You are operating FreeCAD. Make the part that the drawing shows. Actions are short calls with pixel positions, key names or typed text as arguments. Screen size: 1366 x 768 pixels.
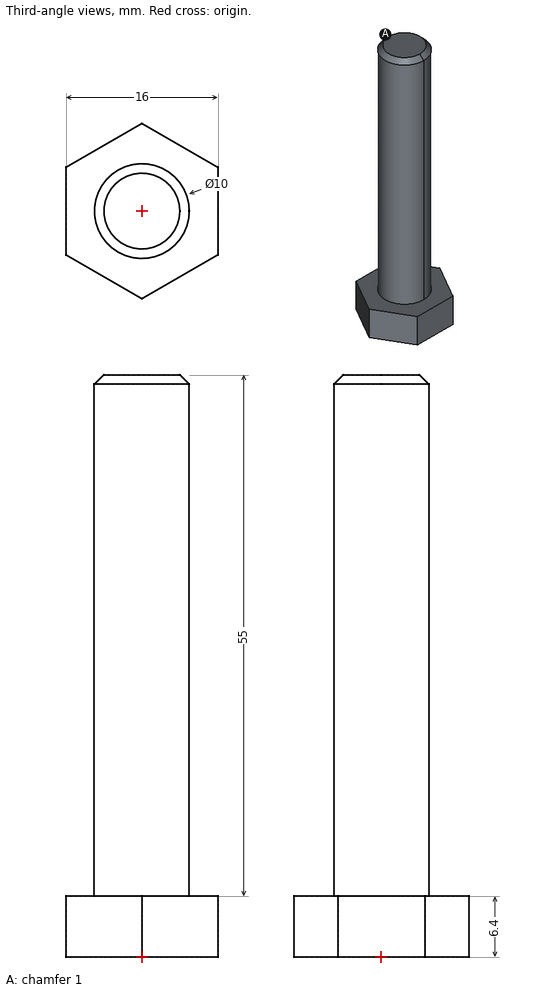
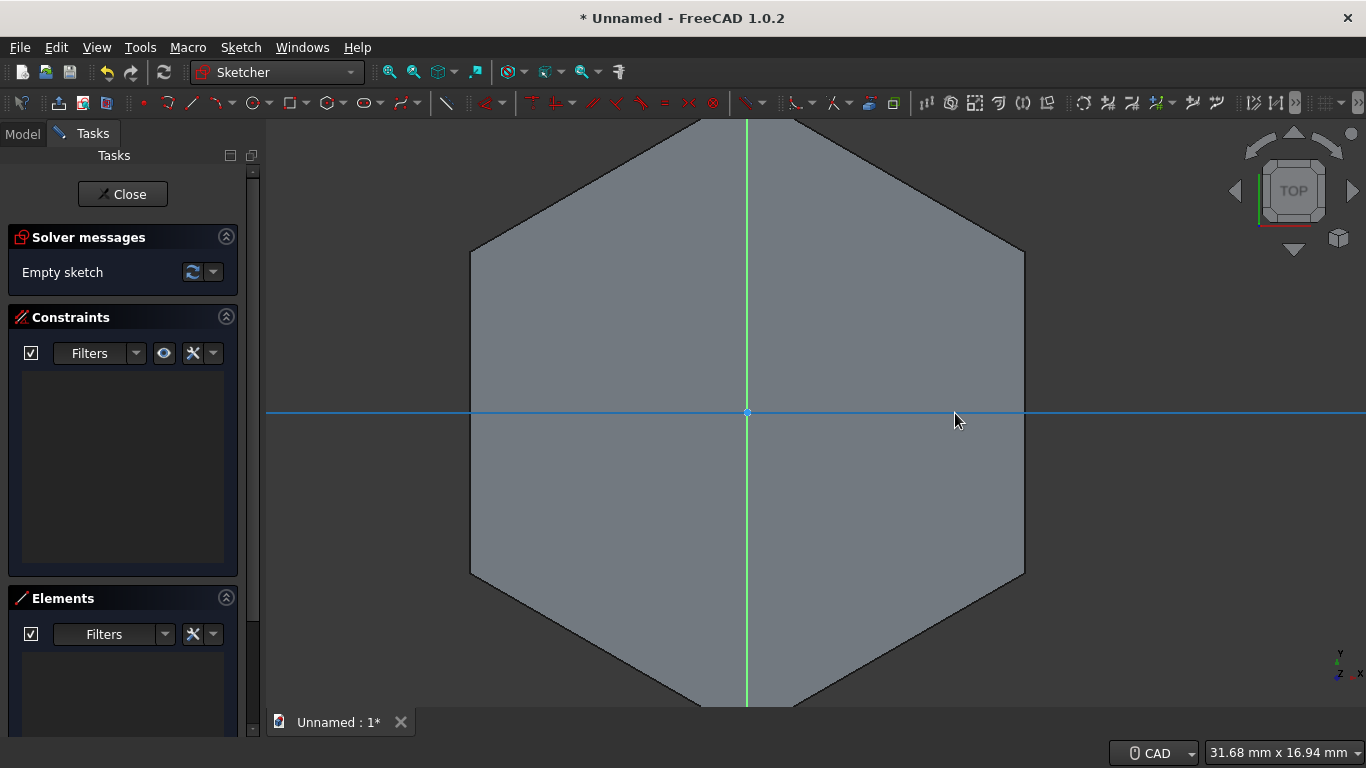
click(254, 104)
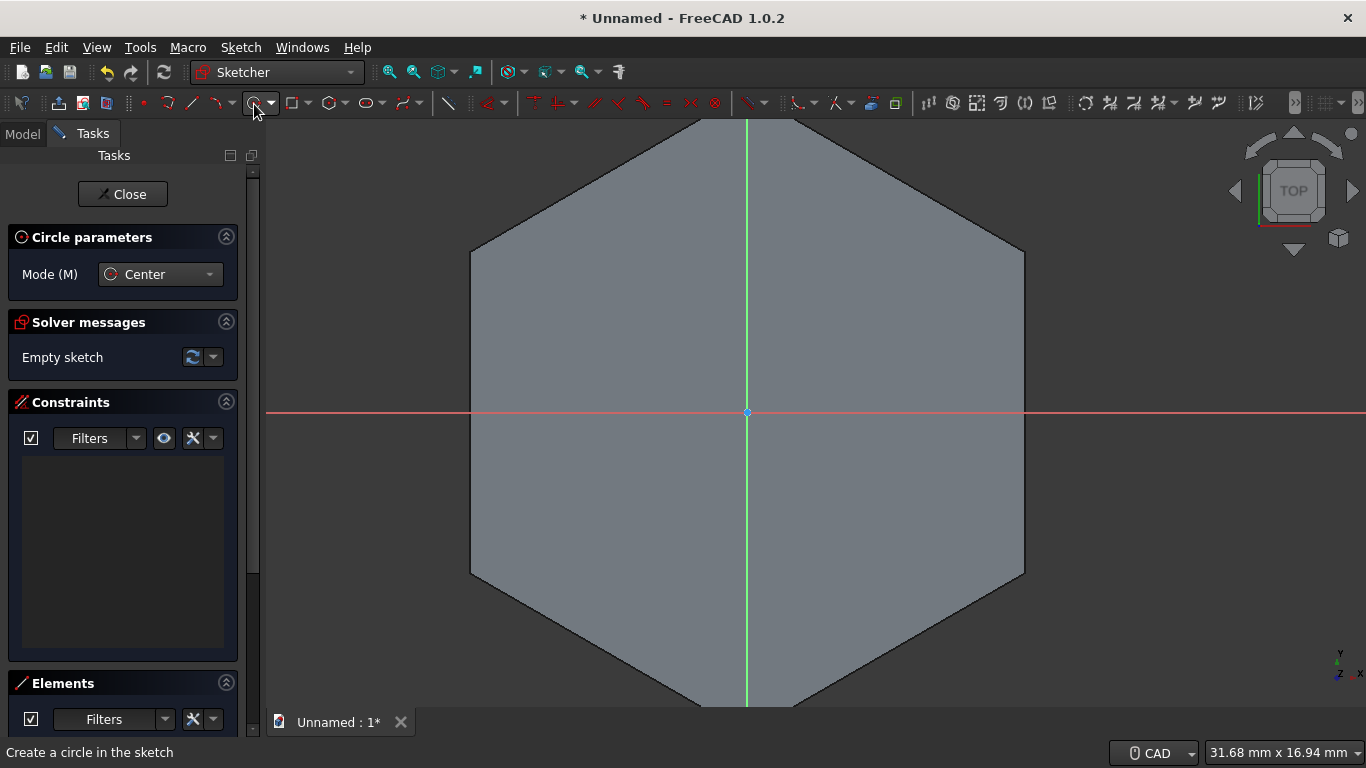
click(747, 413)
move(870, 290)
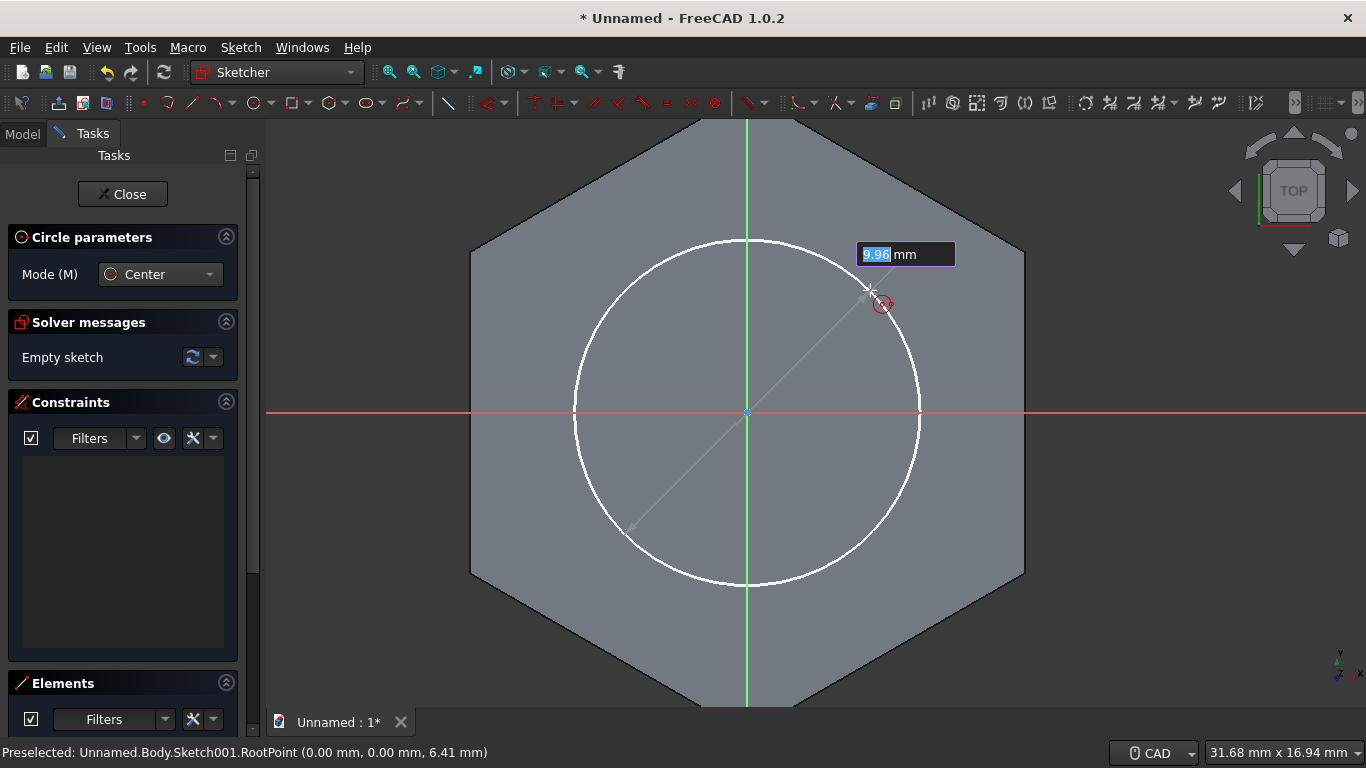
text(10)
key(Return)
key(Escape)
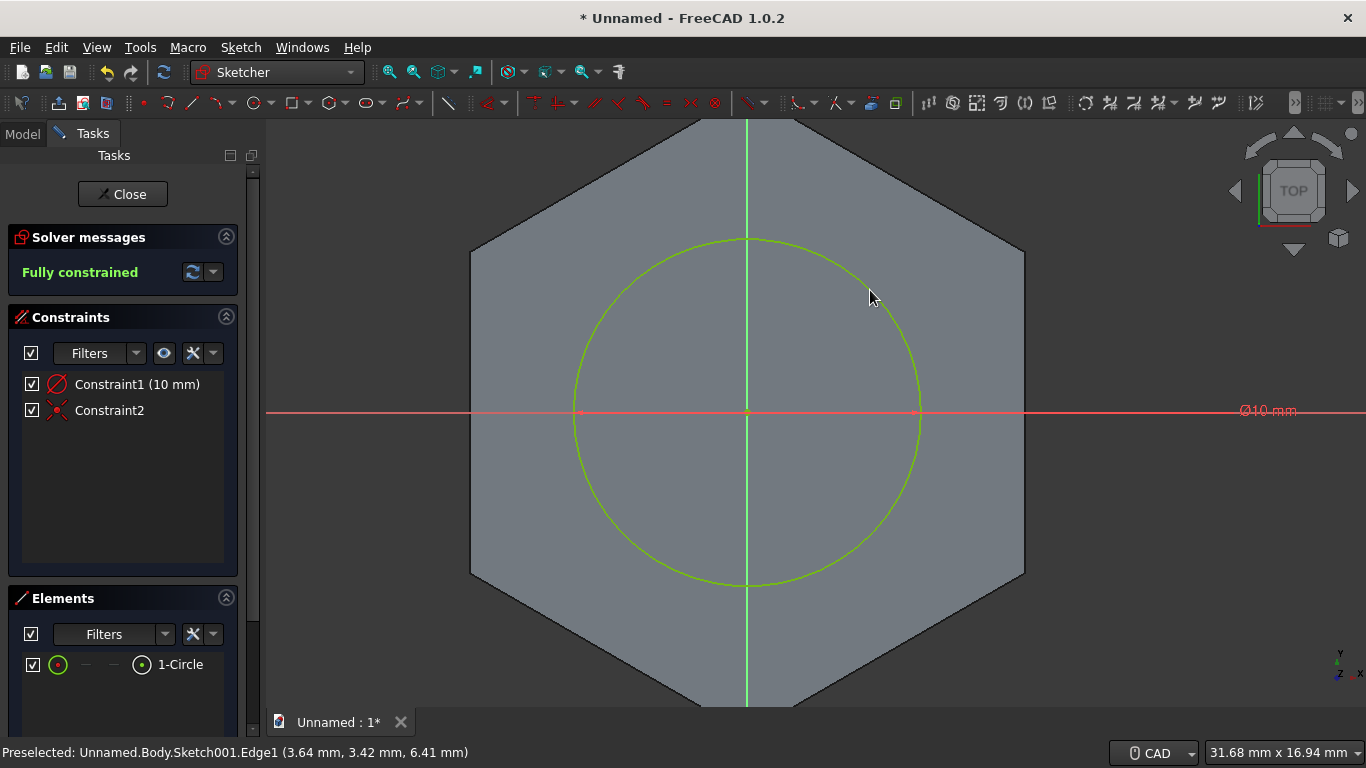
click(123, 194)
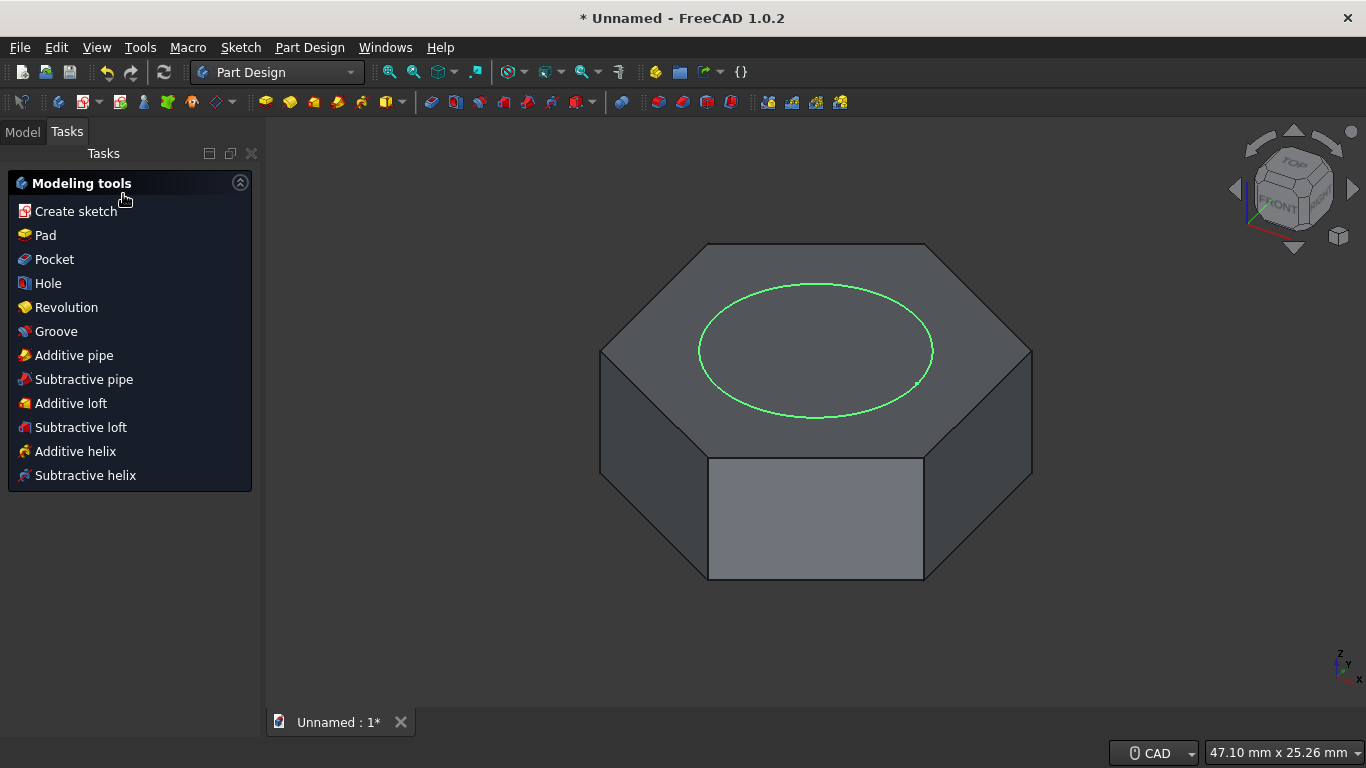
click(266, 102)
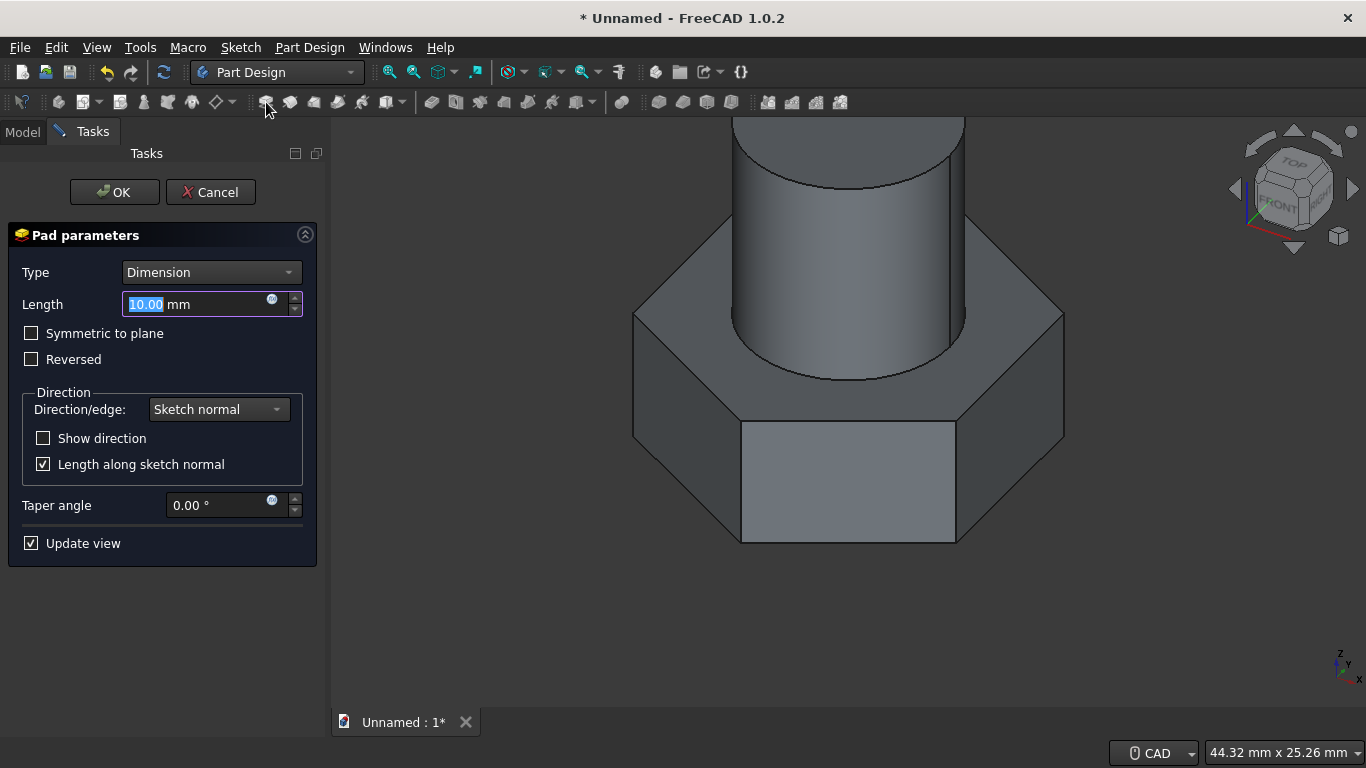
text(55)
key(Tab)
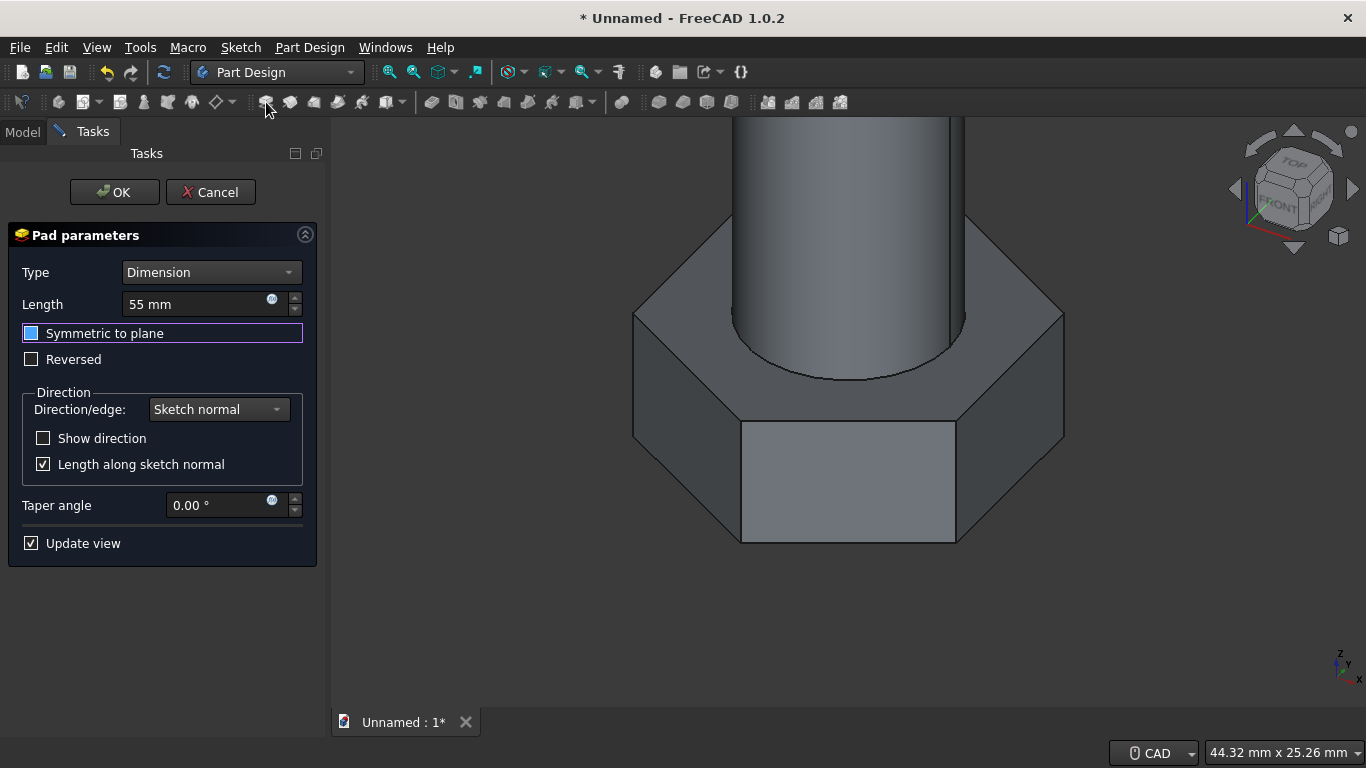
click(115, 192)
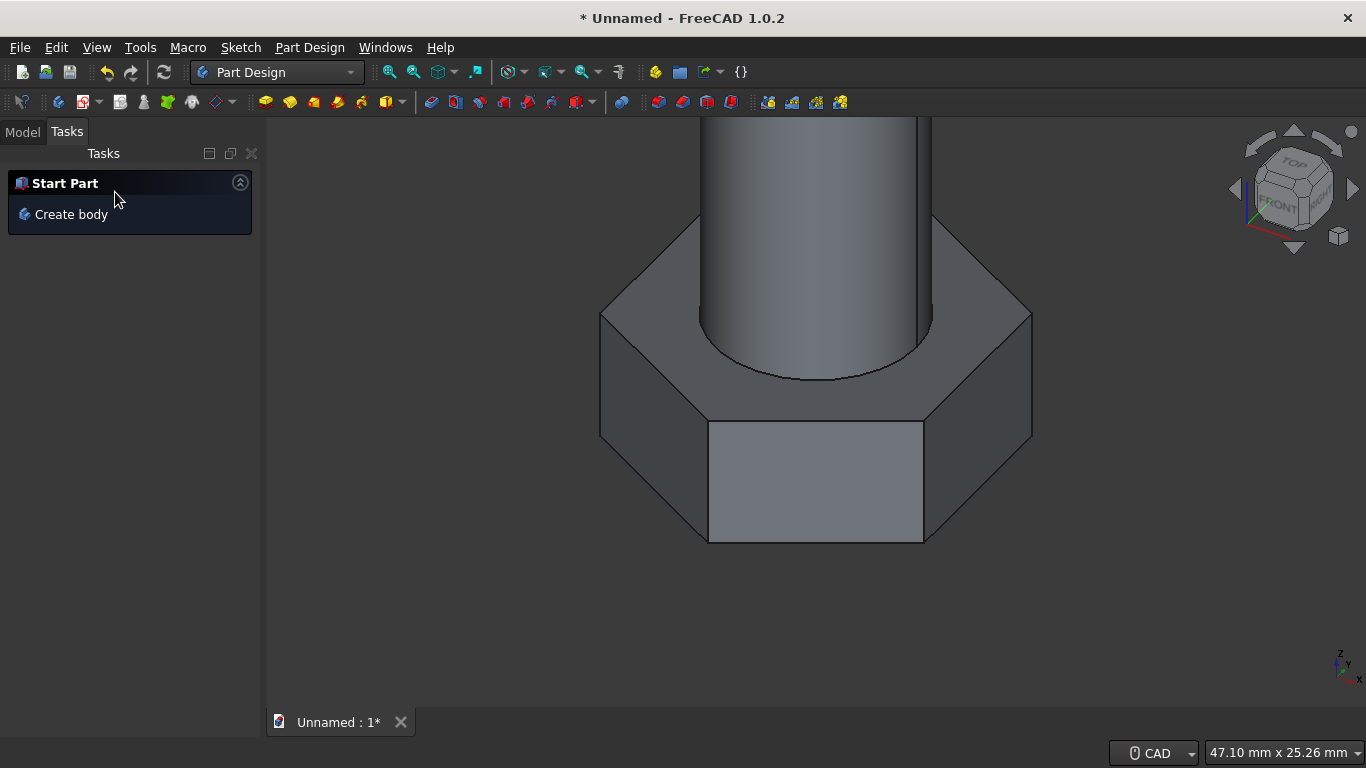
click(390, 72)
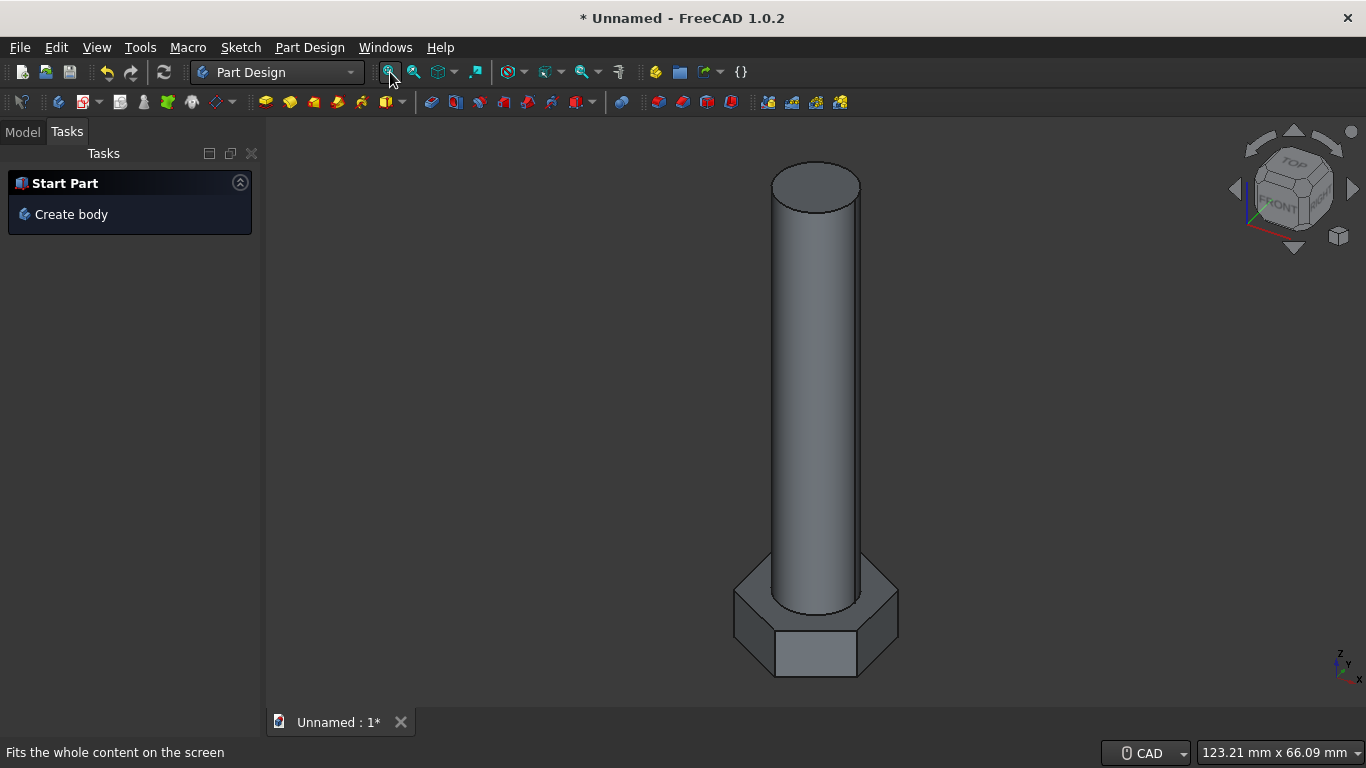
click(772, 189)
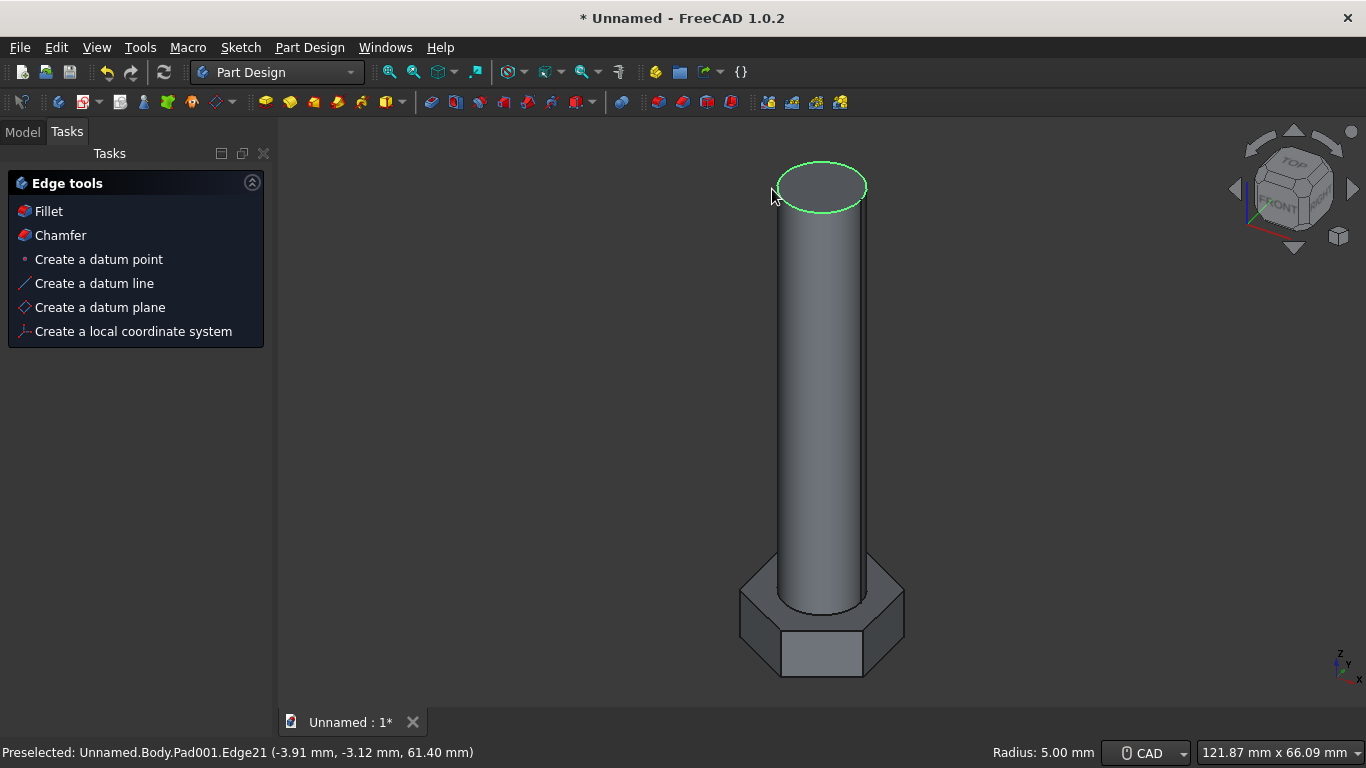
click(684, 102)